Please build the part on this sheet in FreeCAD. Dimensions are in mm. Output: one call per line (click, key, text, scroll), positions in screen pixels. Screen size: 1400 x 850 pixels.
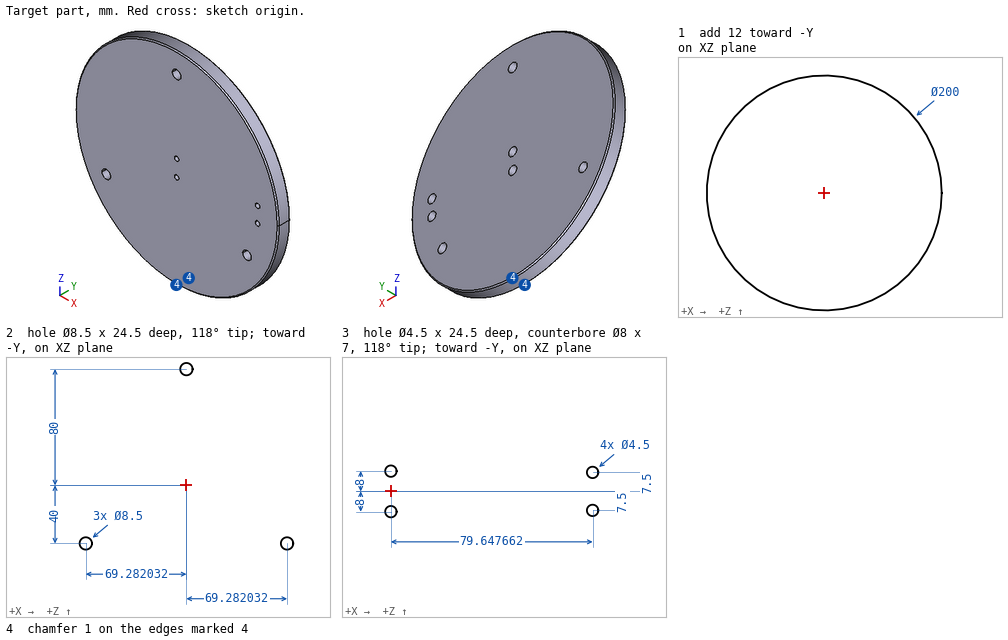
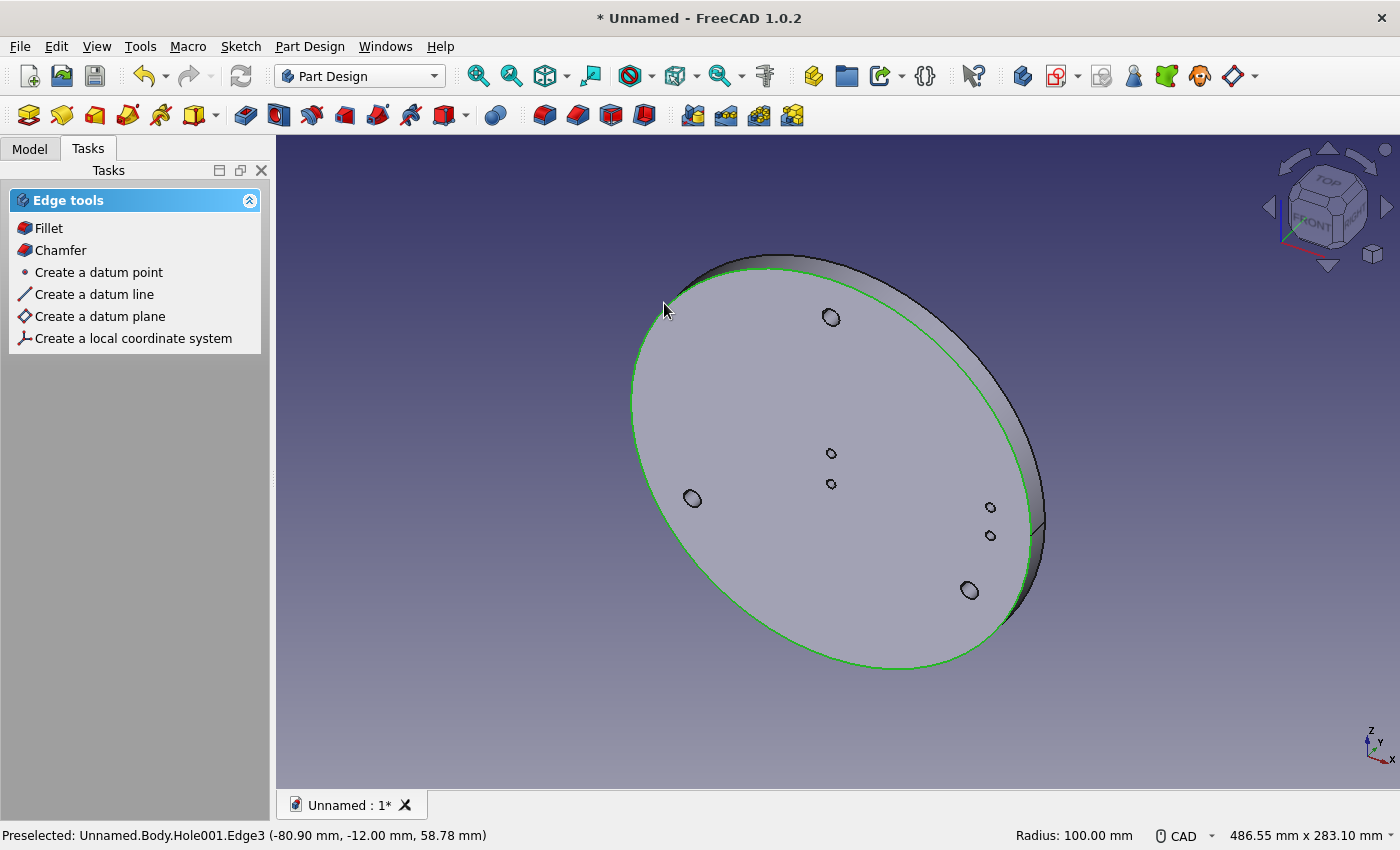
key(0)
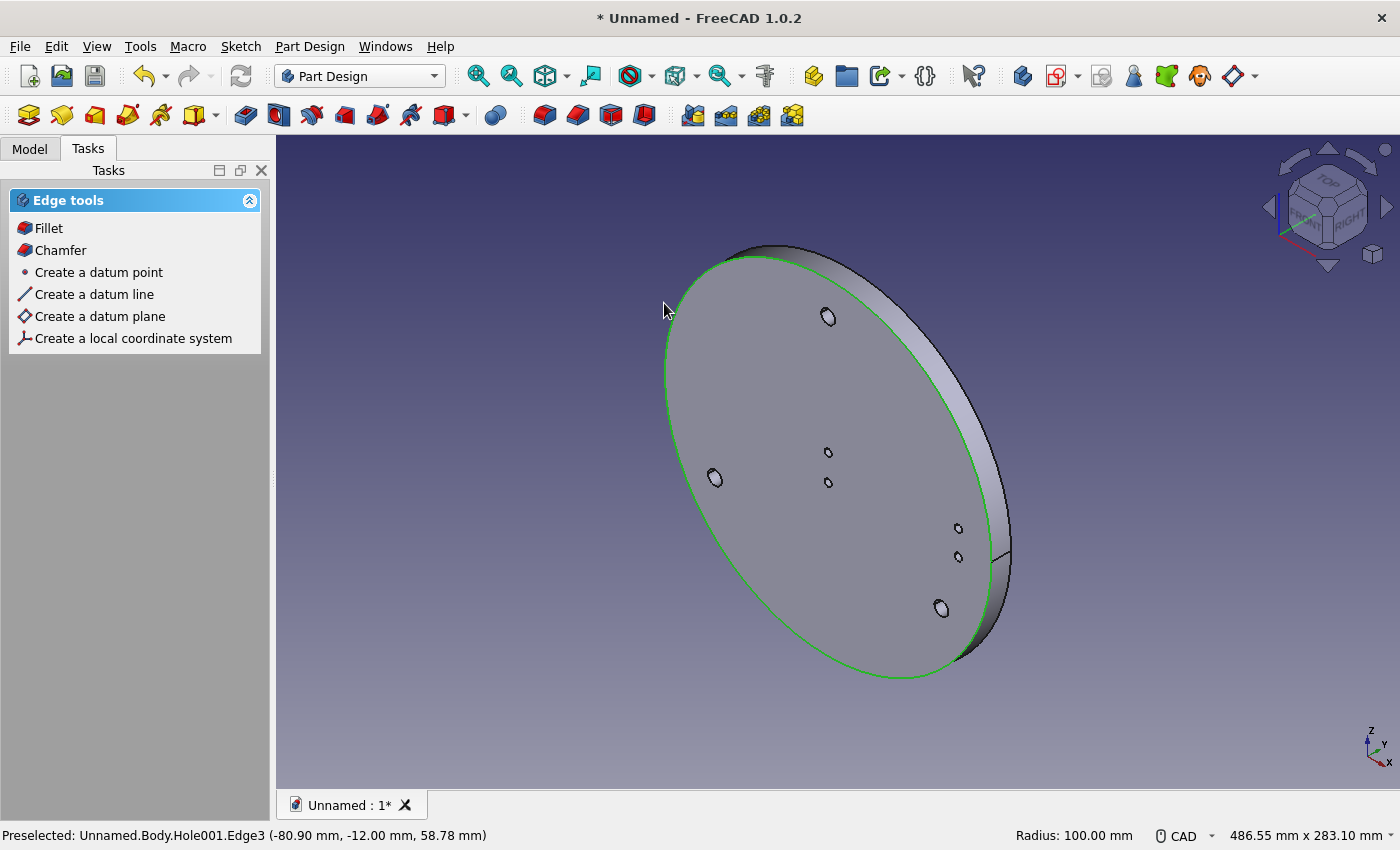
key(2)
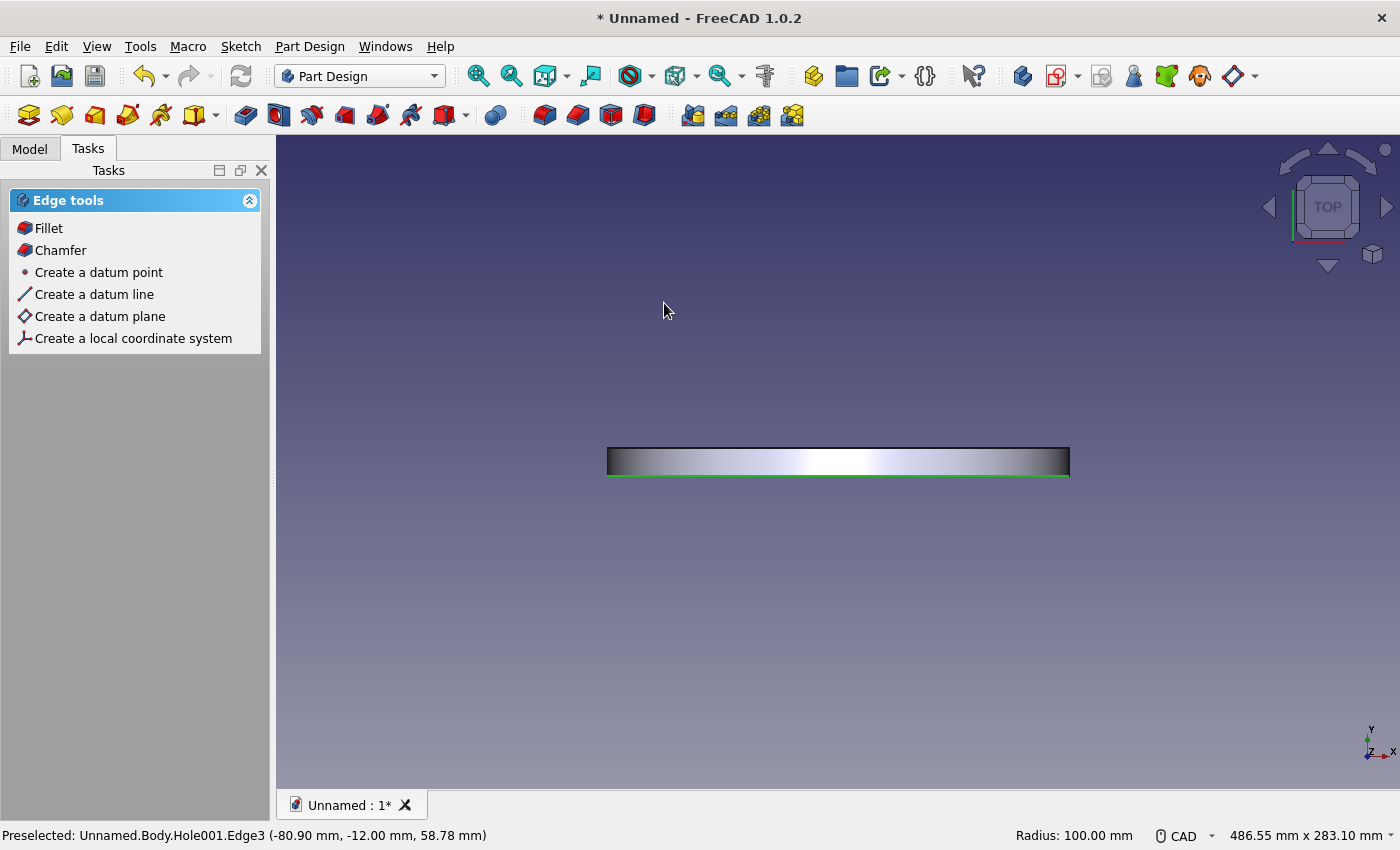
key(v)
key(f)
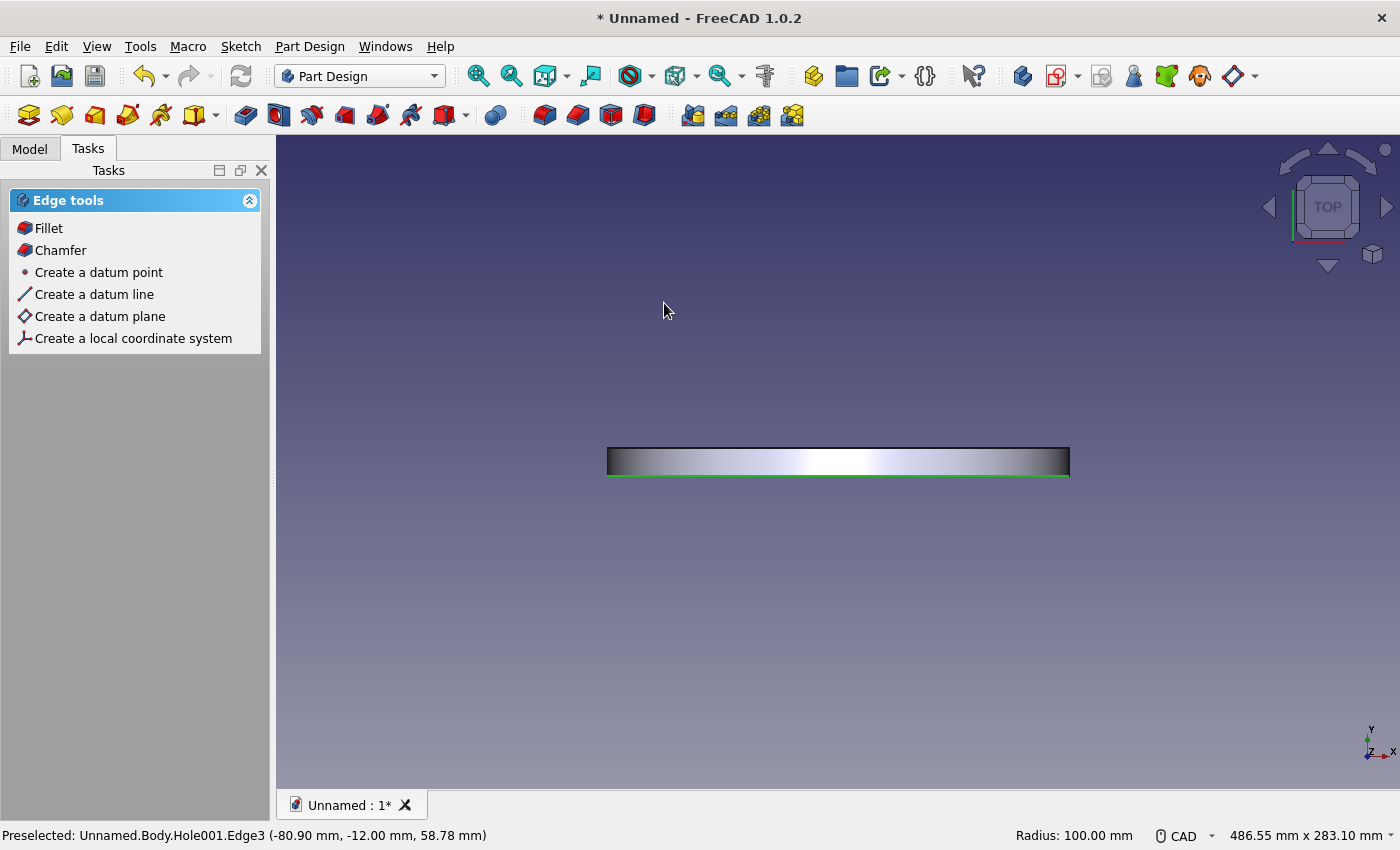
click(651, 447, ctrl)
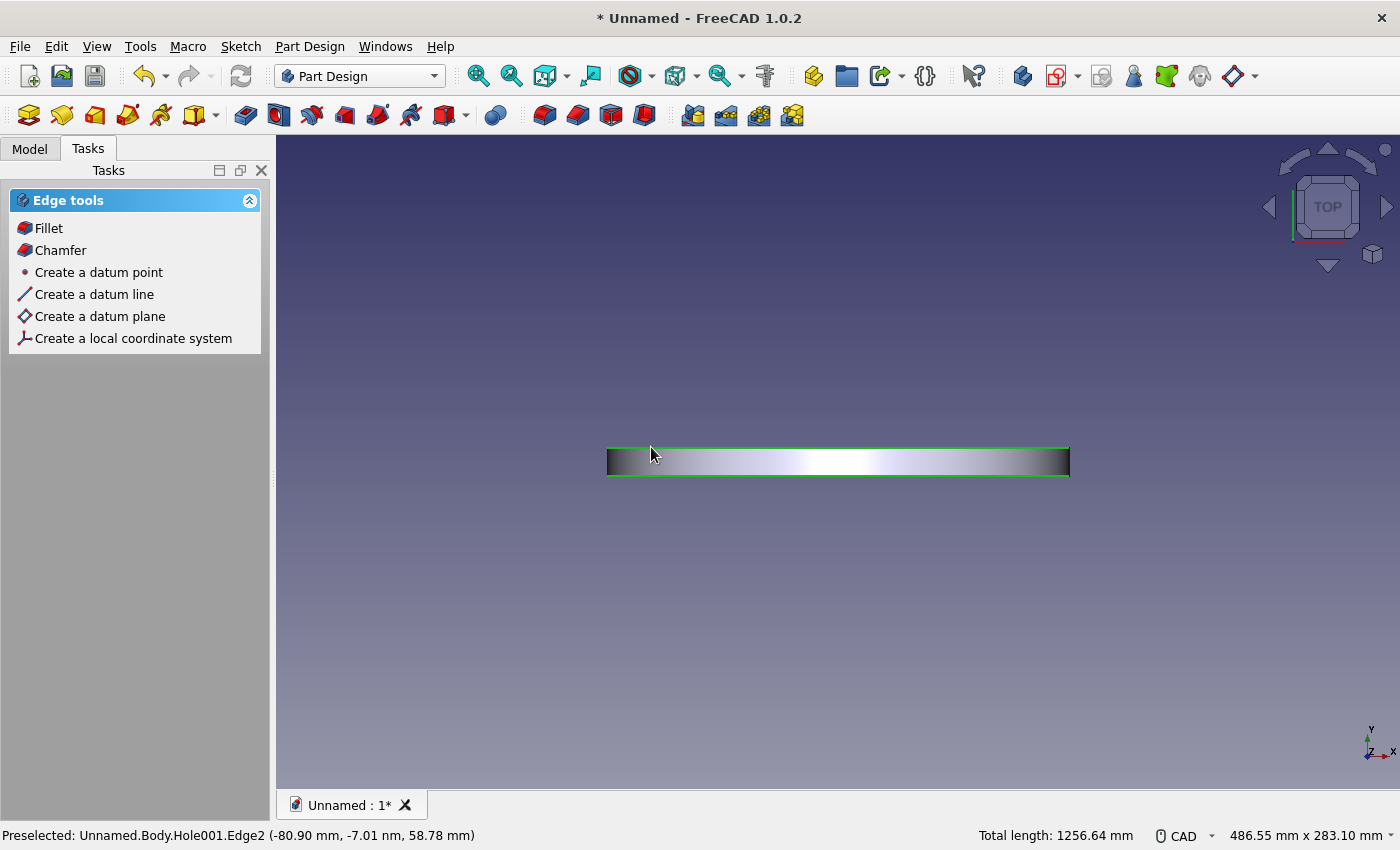
click(578, 116)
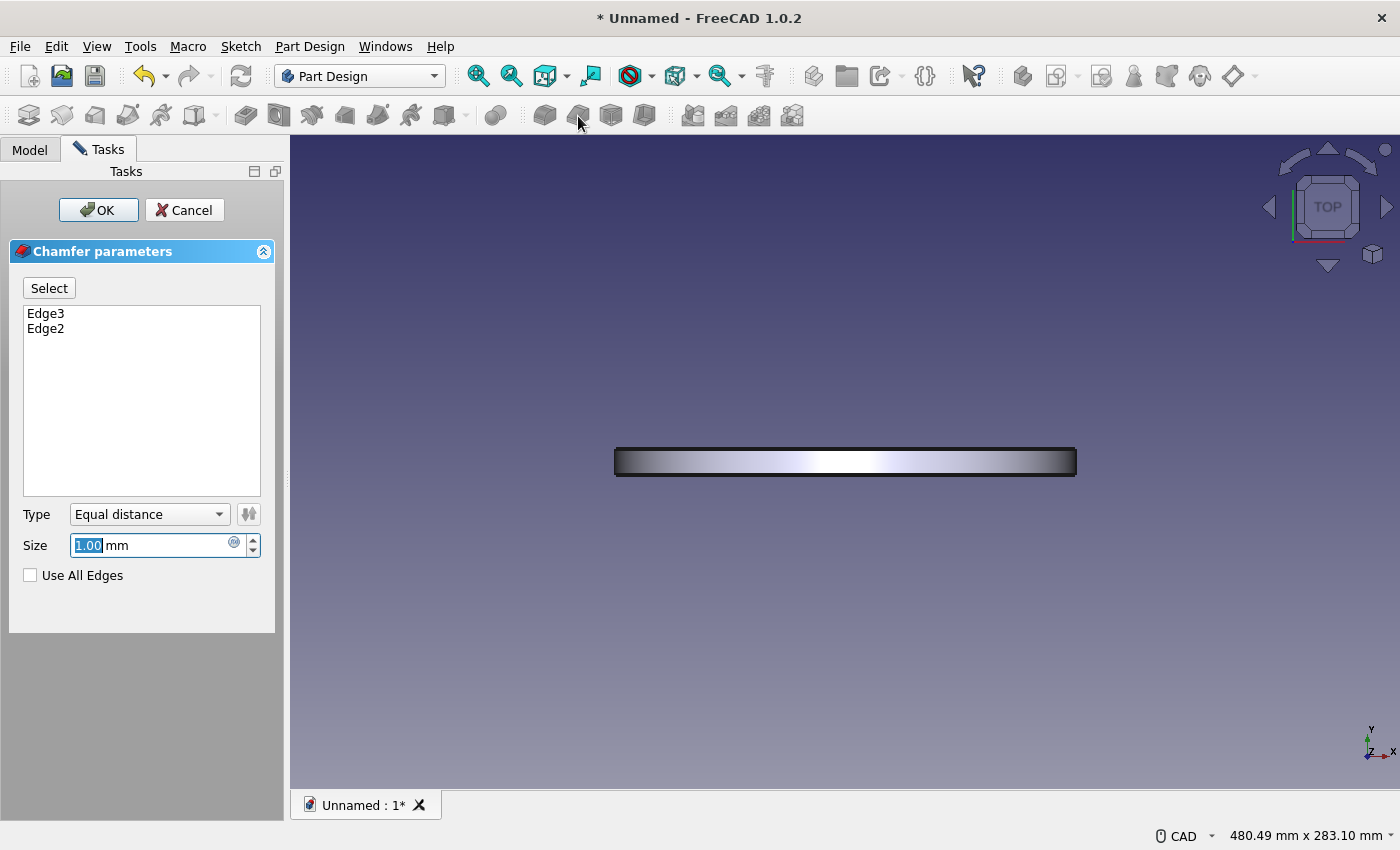
text(1)
key(Tab)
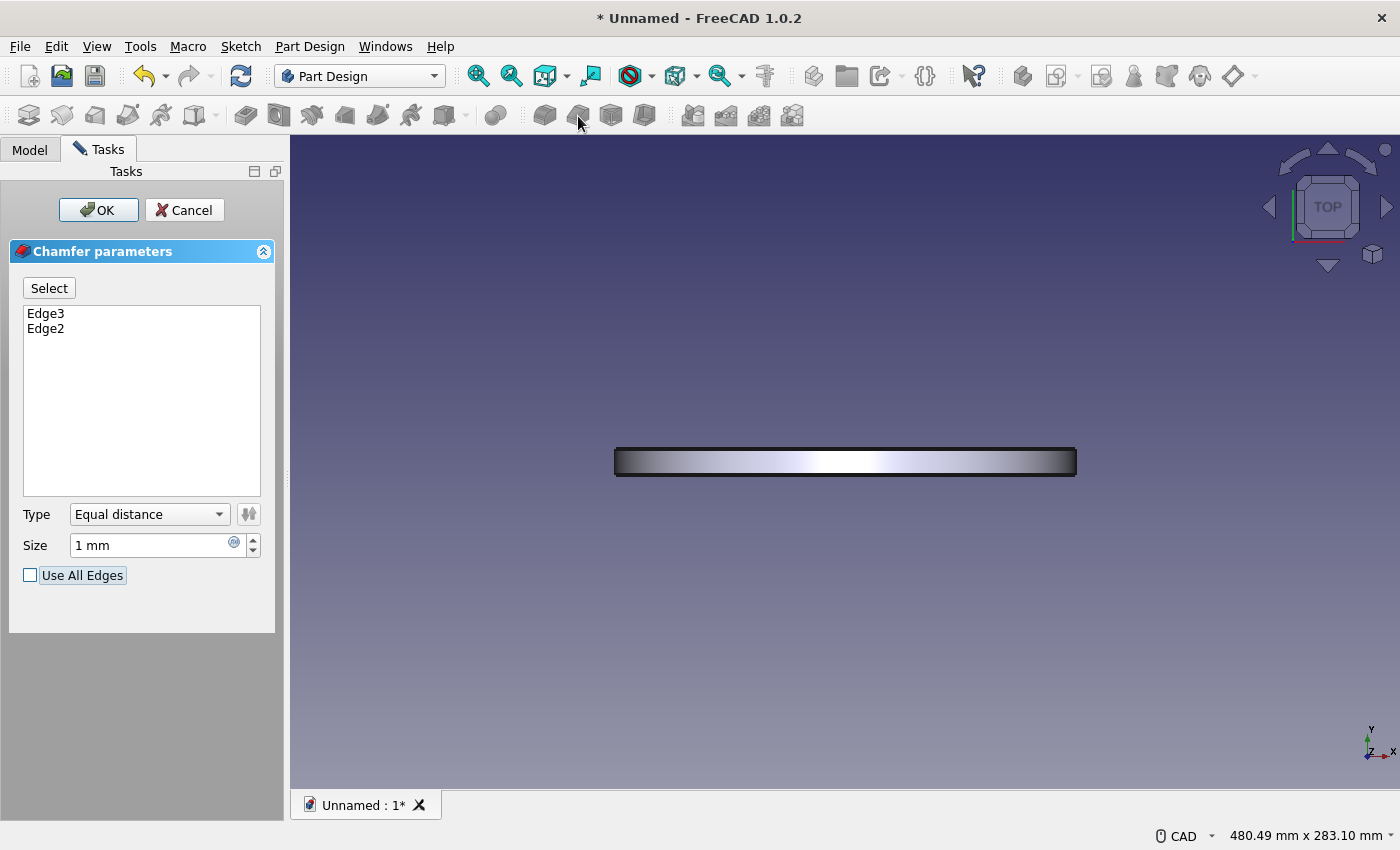
click(99, 210)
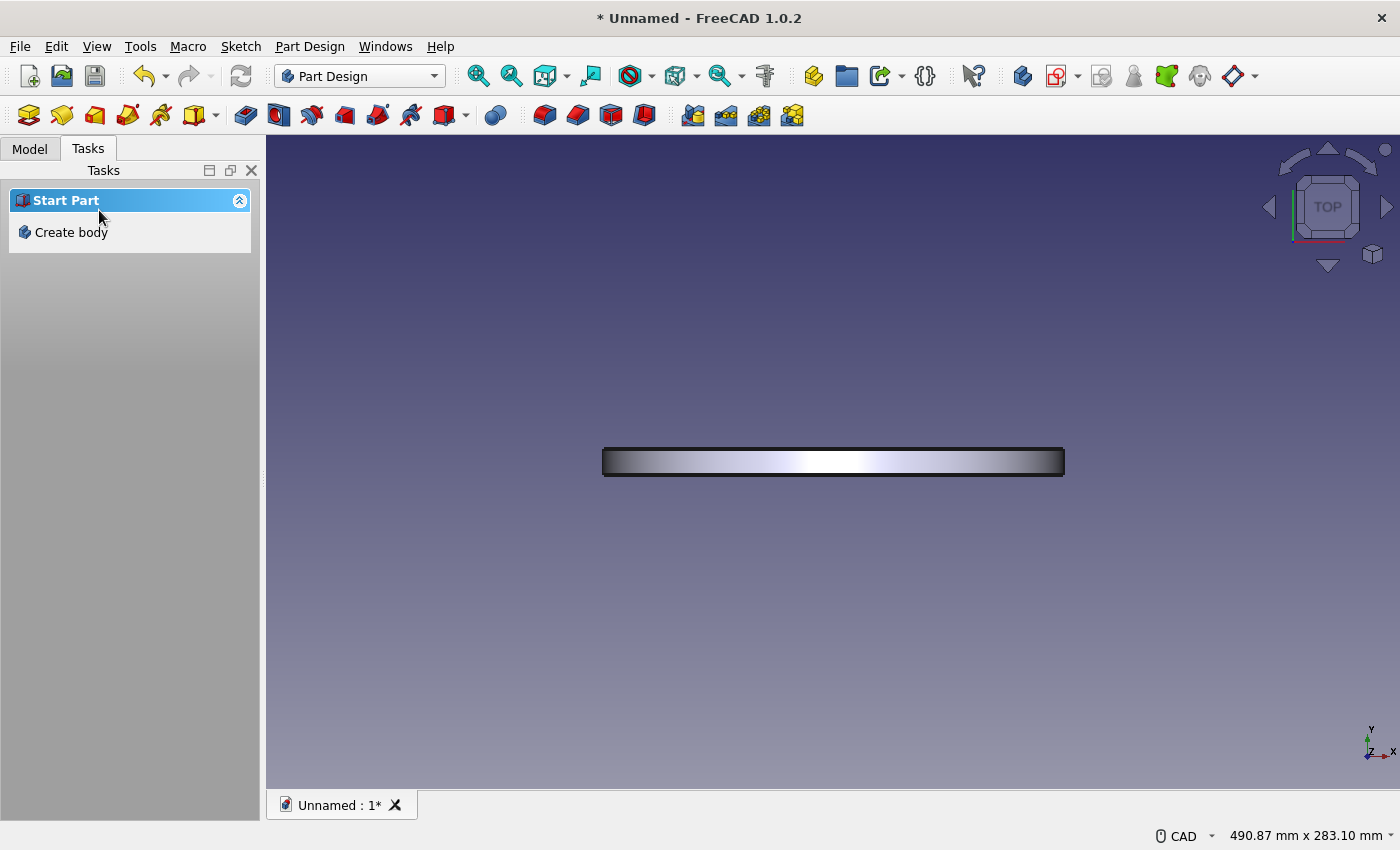
key(0)